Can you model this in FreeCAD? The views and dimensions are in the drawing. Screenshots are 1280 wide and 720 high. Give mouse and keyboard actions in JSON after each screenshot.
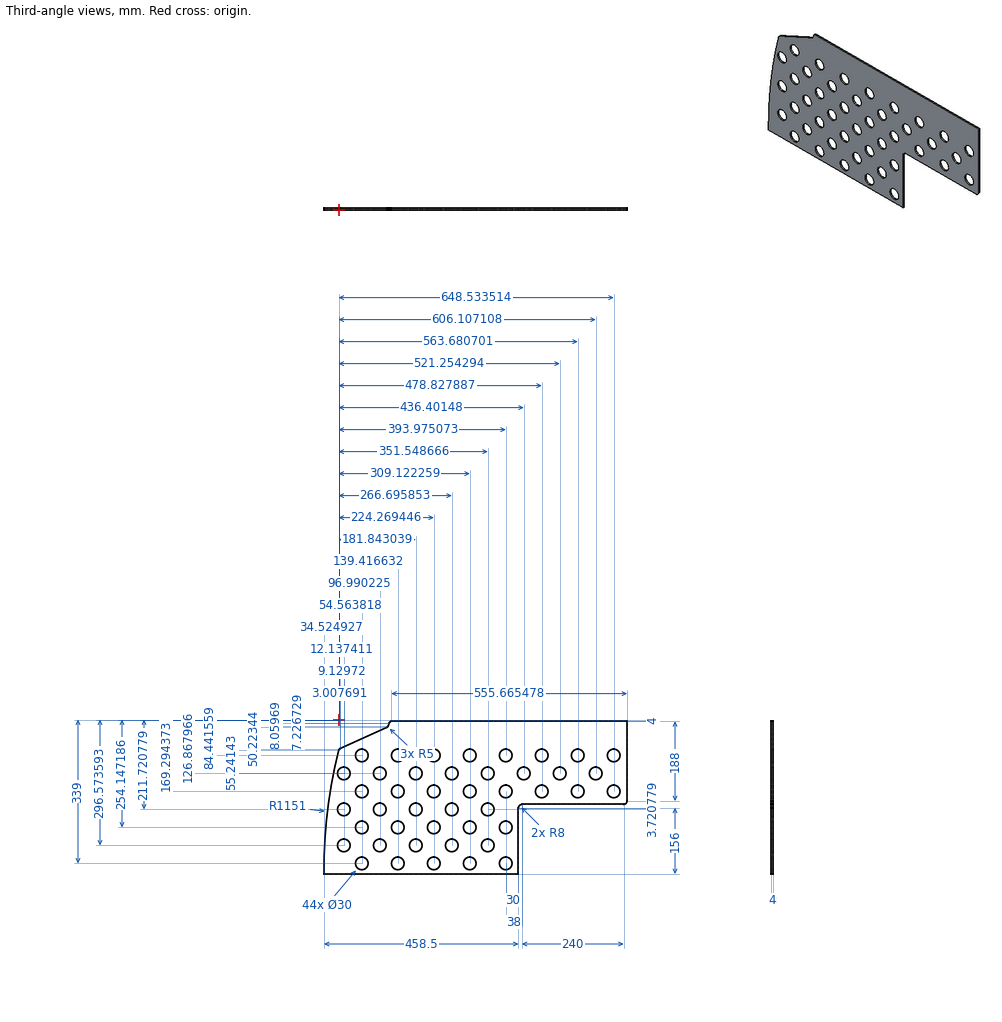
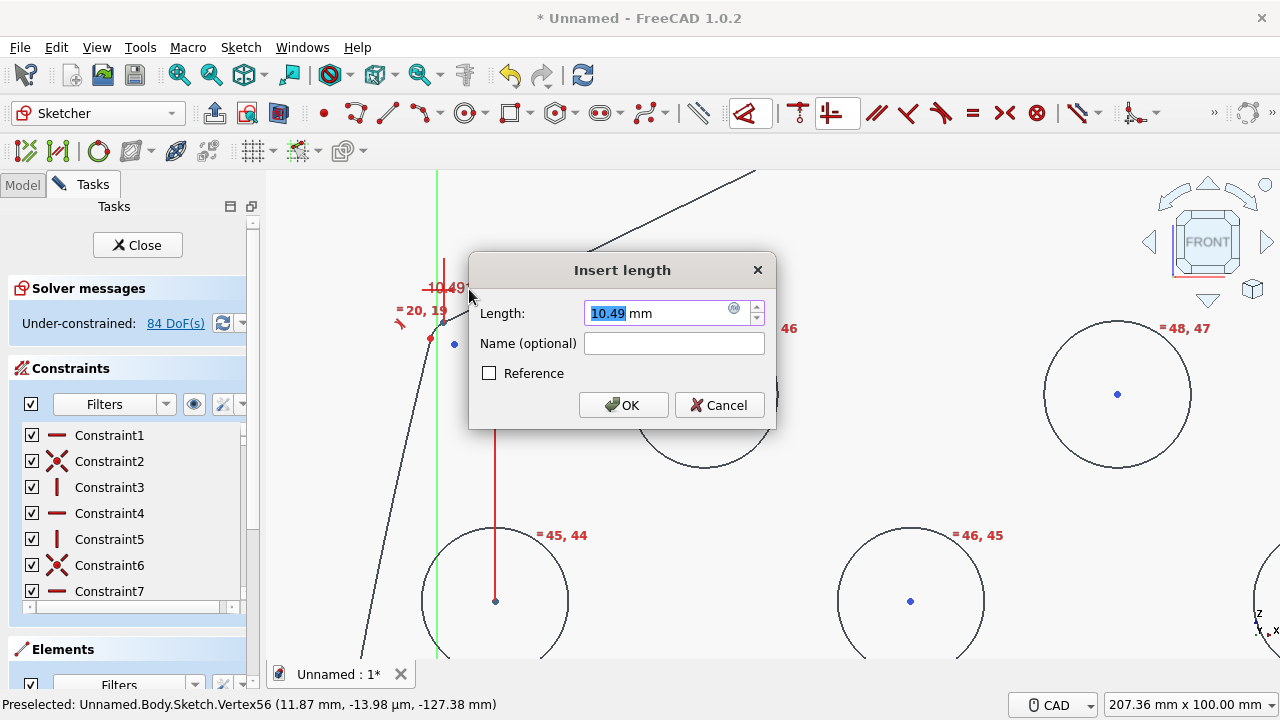
{"action": "type", "text": "9.12972"}
{"action": "key", "text": "Return"}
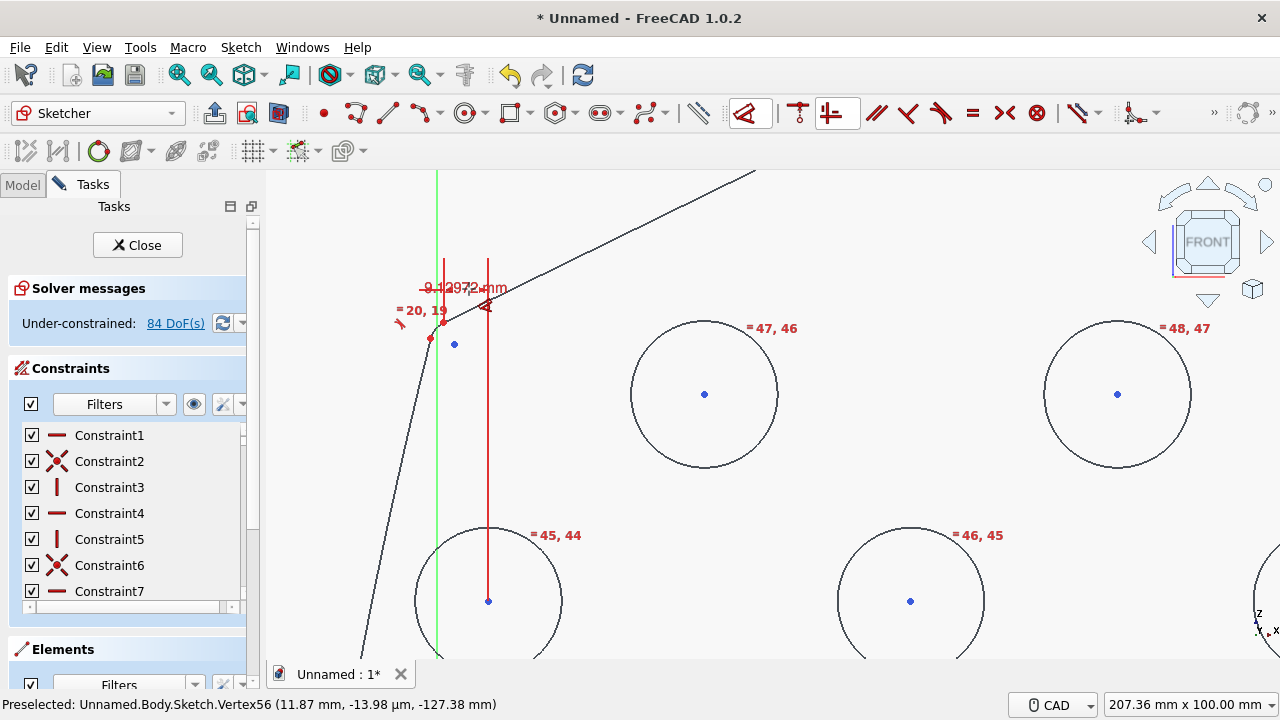
{"action": "scroll", "coordinate": [445, 325], "scroll_direction": "down", "scroll_amount": 9}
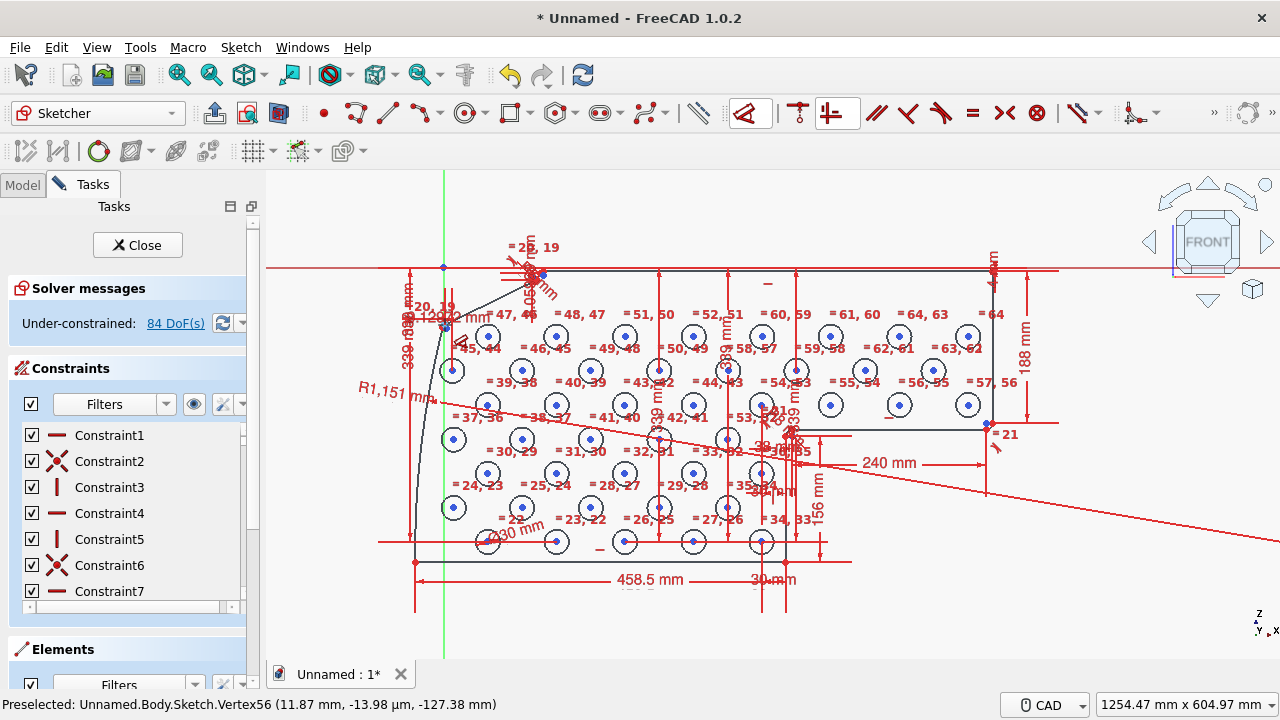
{"action": "scroll", "coordinate": [540, 273], "scroll_direction": "up", "scroll_amount": 10}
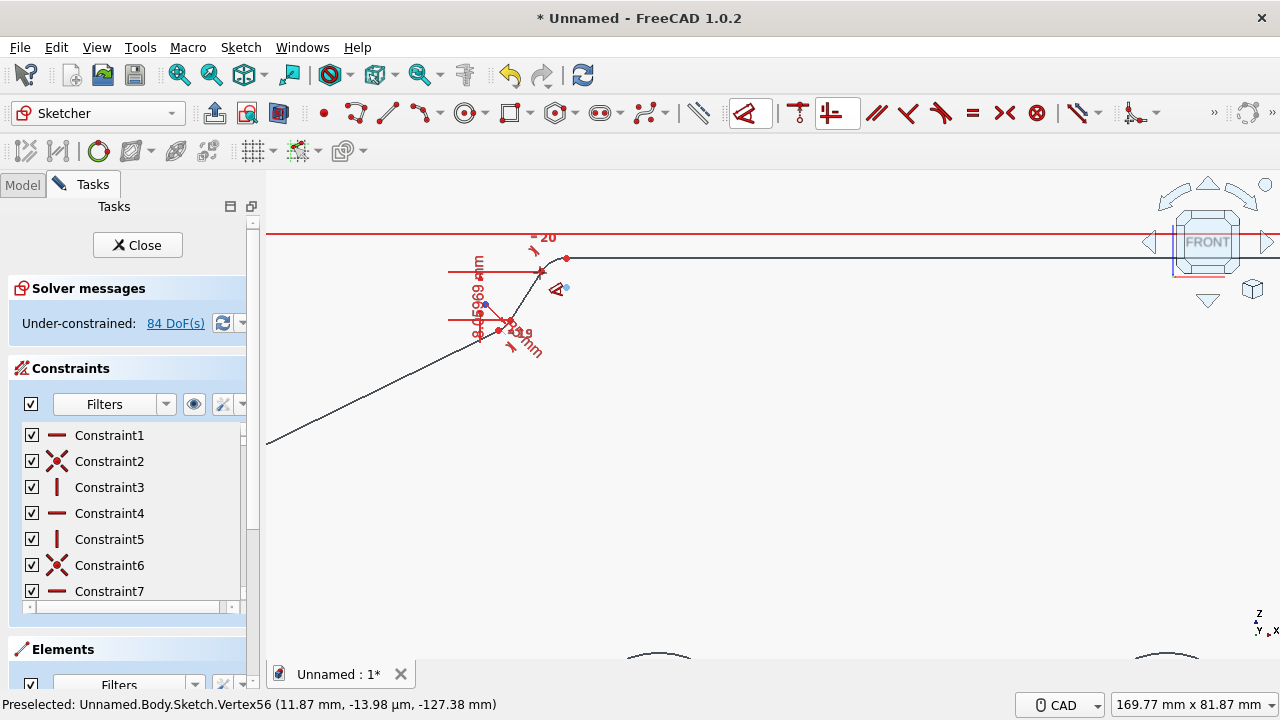
{"action": "left_click", "coordinate": [541, 272]}
{"action": "left_click", "coordinate": [575, 244]}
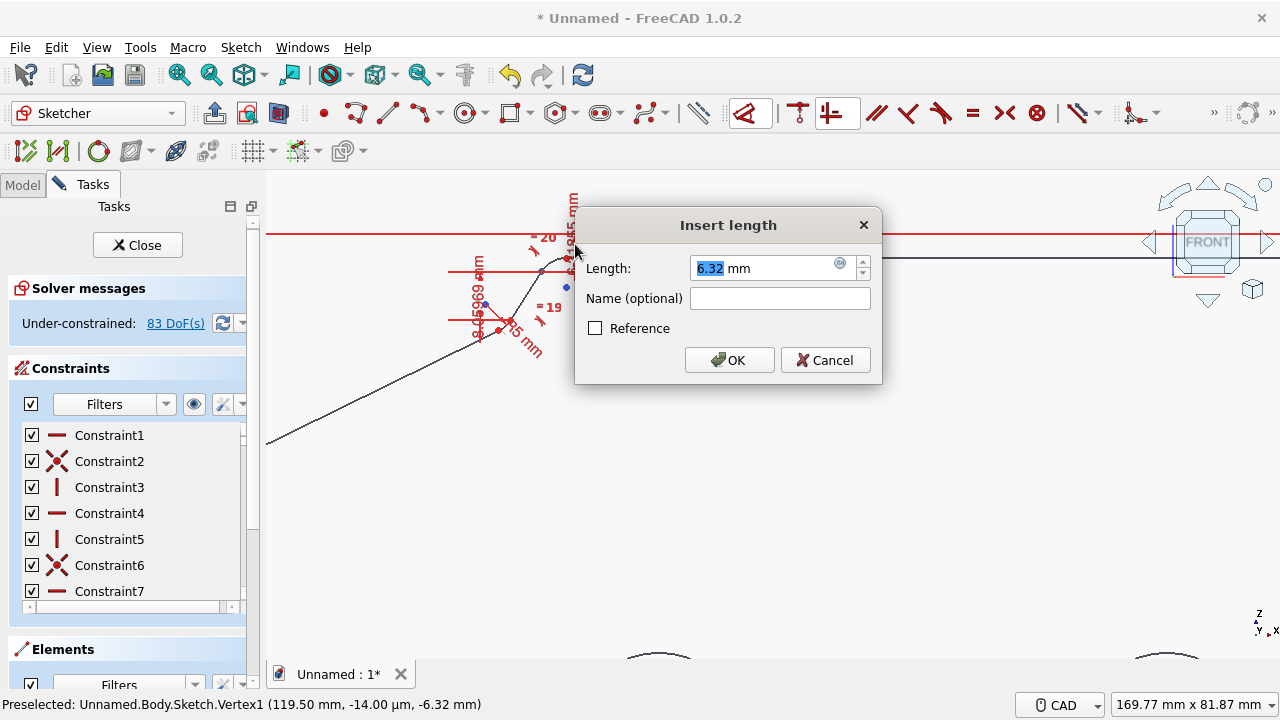
{"action": "type", "text": "7.226729"}
{"action": "key", "text": "Return"}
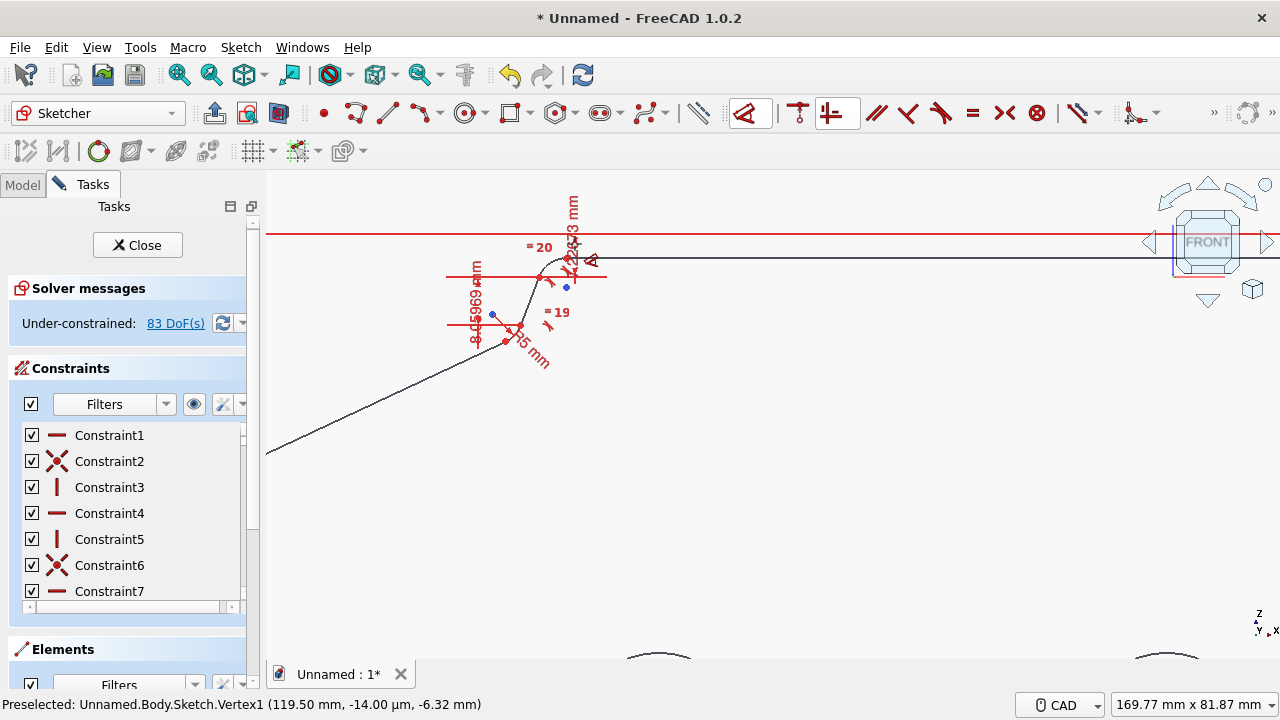
{"action": "scroll", "coordinate": [540, 273], "scroll_direction": "down", "scroll_amount": 10}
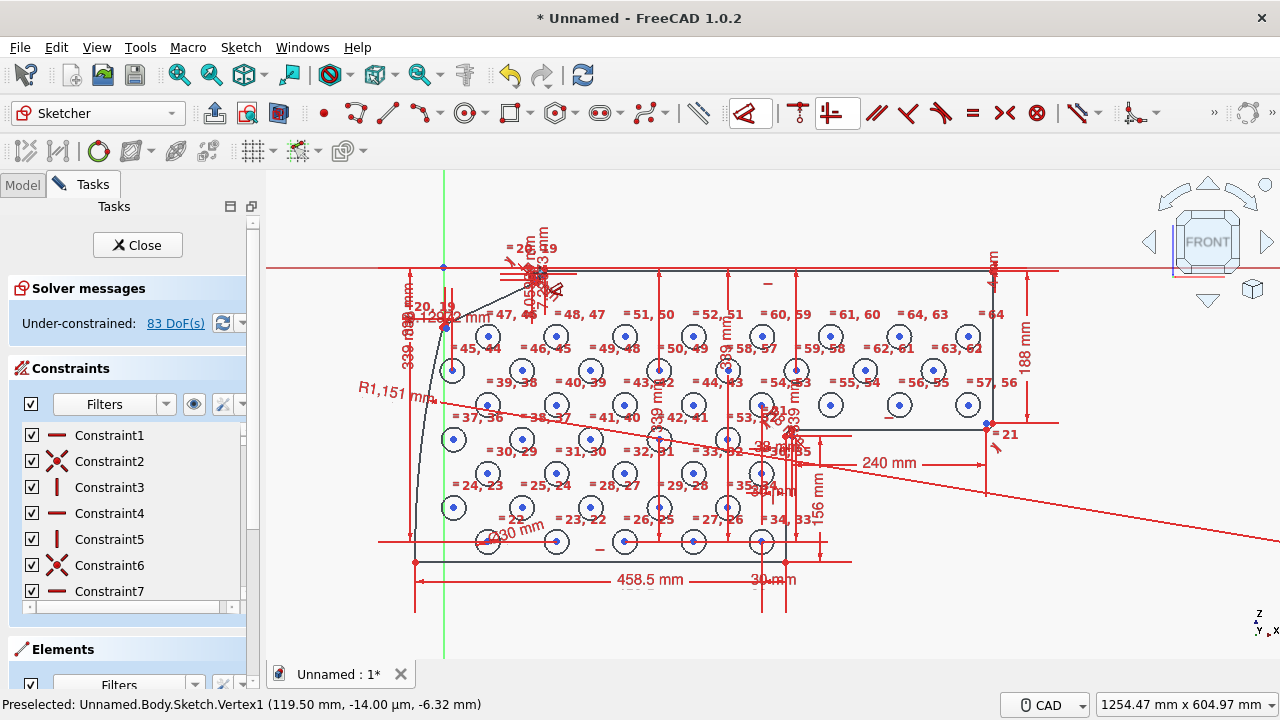
{"action": "scroll", "coordinate": [445, 325], "scroll_direction": "up", "scroll_amount": 14}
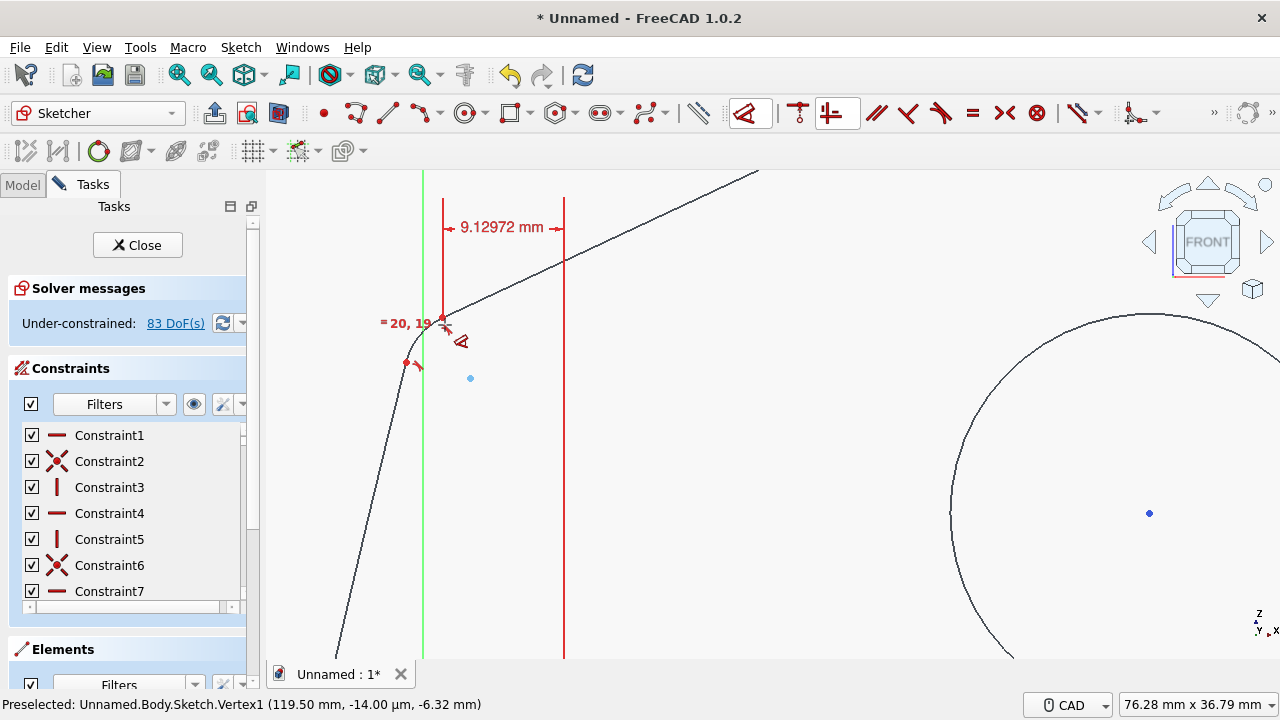
{"action": "left_click", "coordinate": [443, 318]}
{"action": "left_click", "coordinate": [437, 352]}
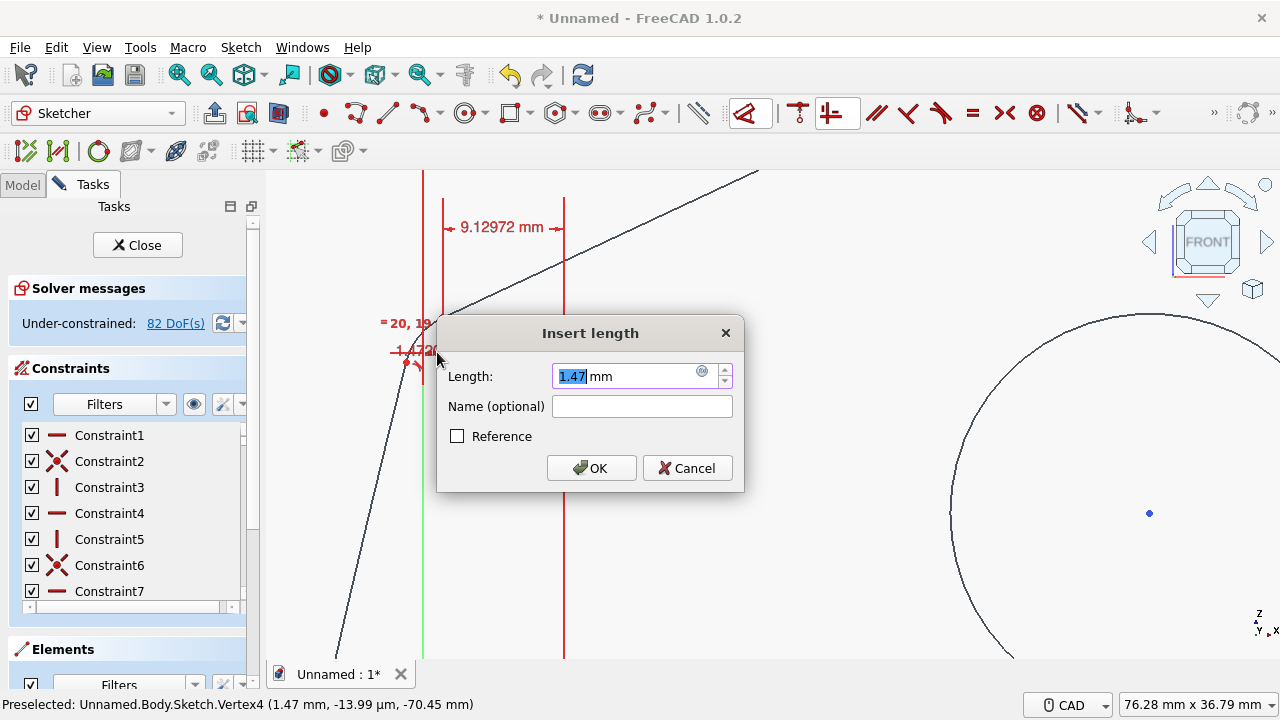
{"action": "type", "text": "3.007691"}
{"action": "key", "text": "Return"}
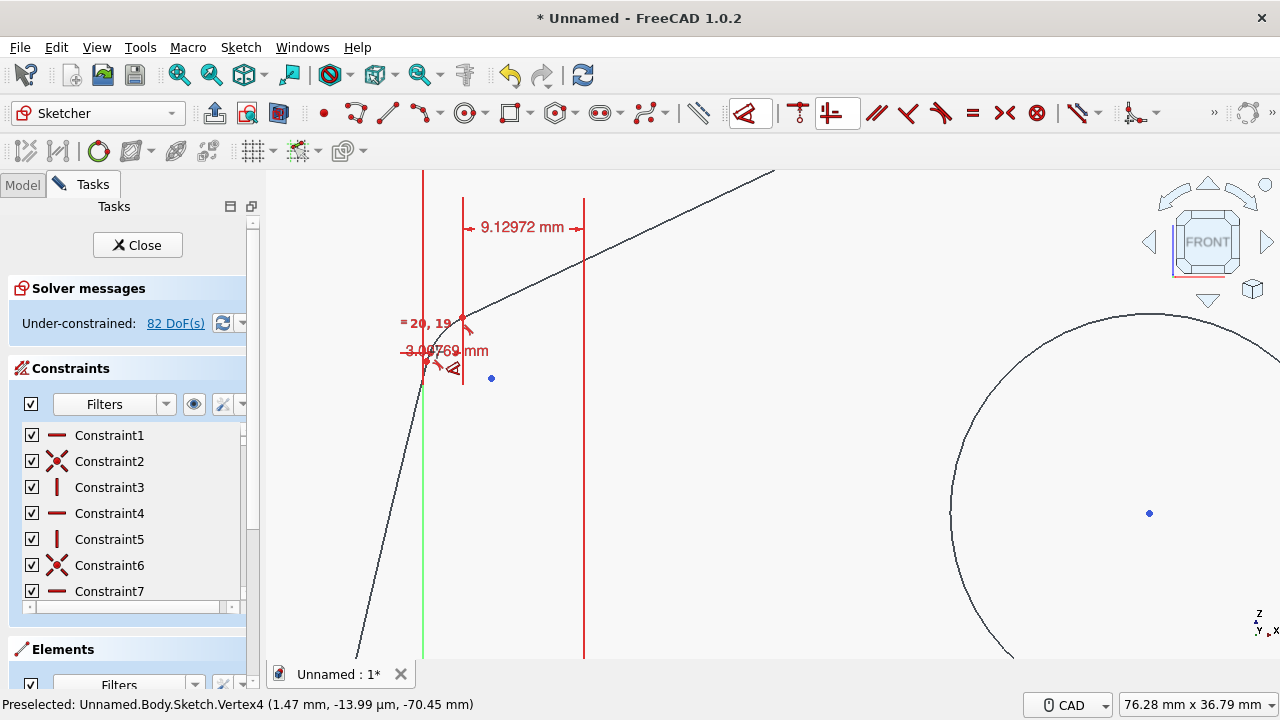
{"action": "scroll", "coordinate": [445, 325], "scroll_direction": "down", "scroll_amount": 14}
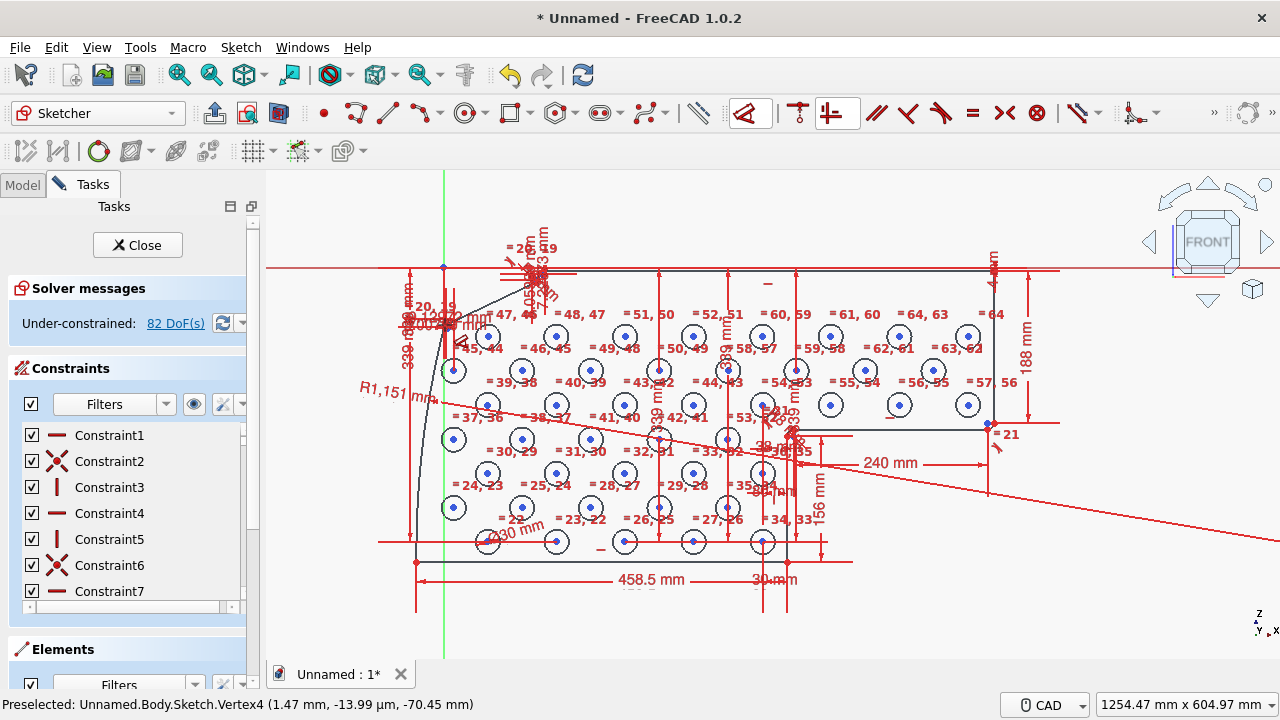
{"action": "left_click", "coordinate": [509, 295]}
{"action": "left_click", "coordinate": [412, 289]}